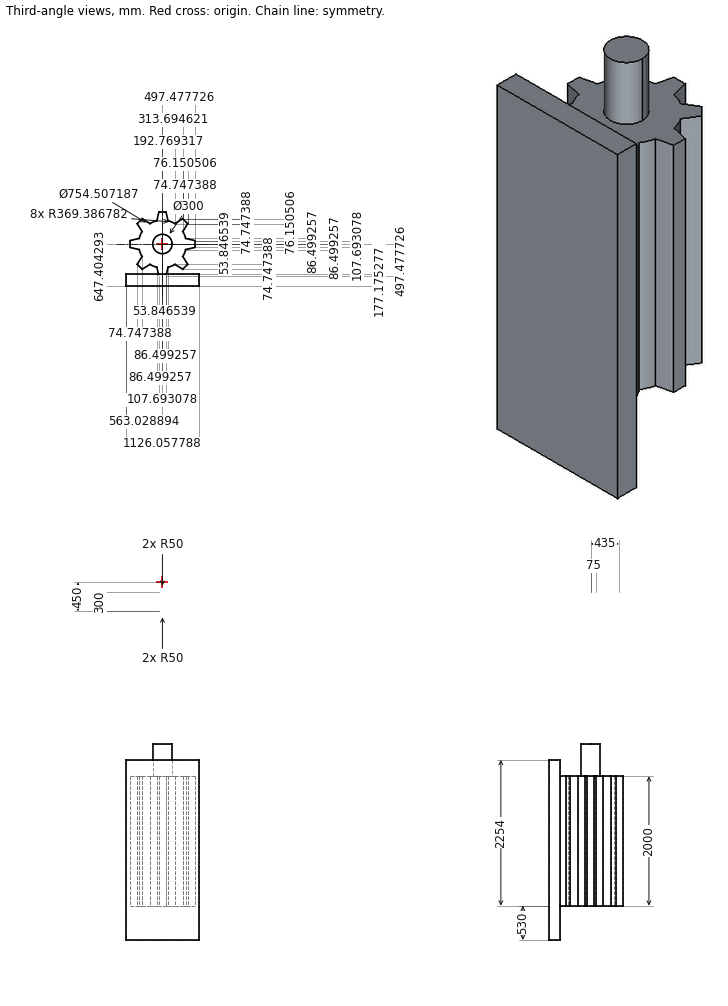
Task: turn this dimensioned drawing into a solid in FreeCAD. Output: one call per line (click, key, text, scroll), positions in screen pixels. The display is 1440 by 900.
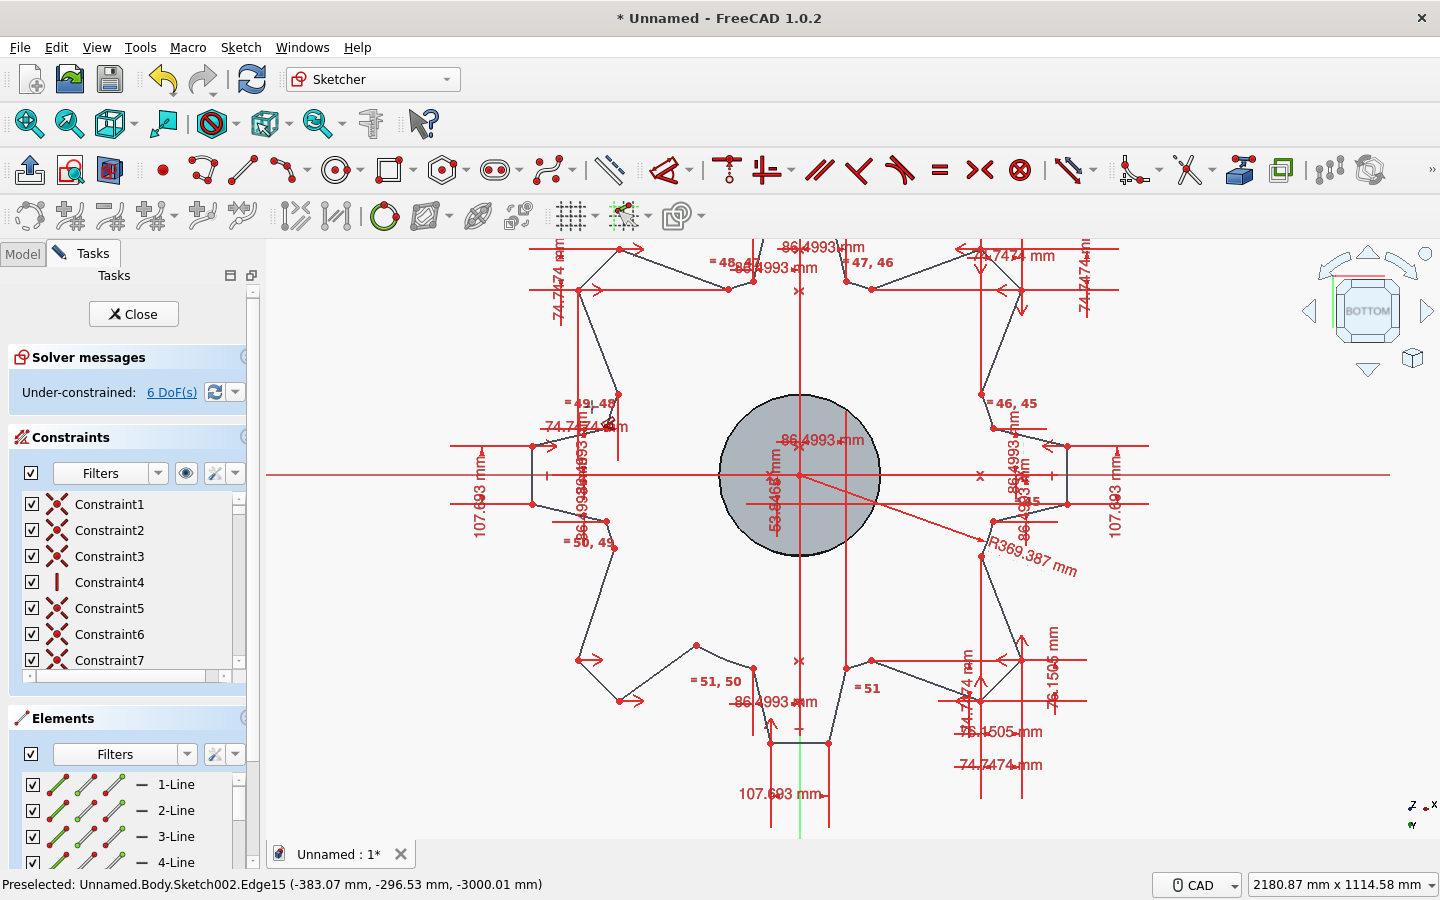
click(604, 582)
click(588, 694)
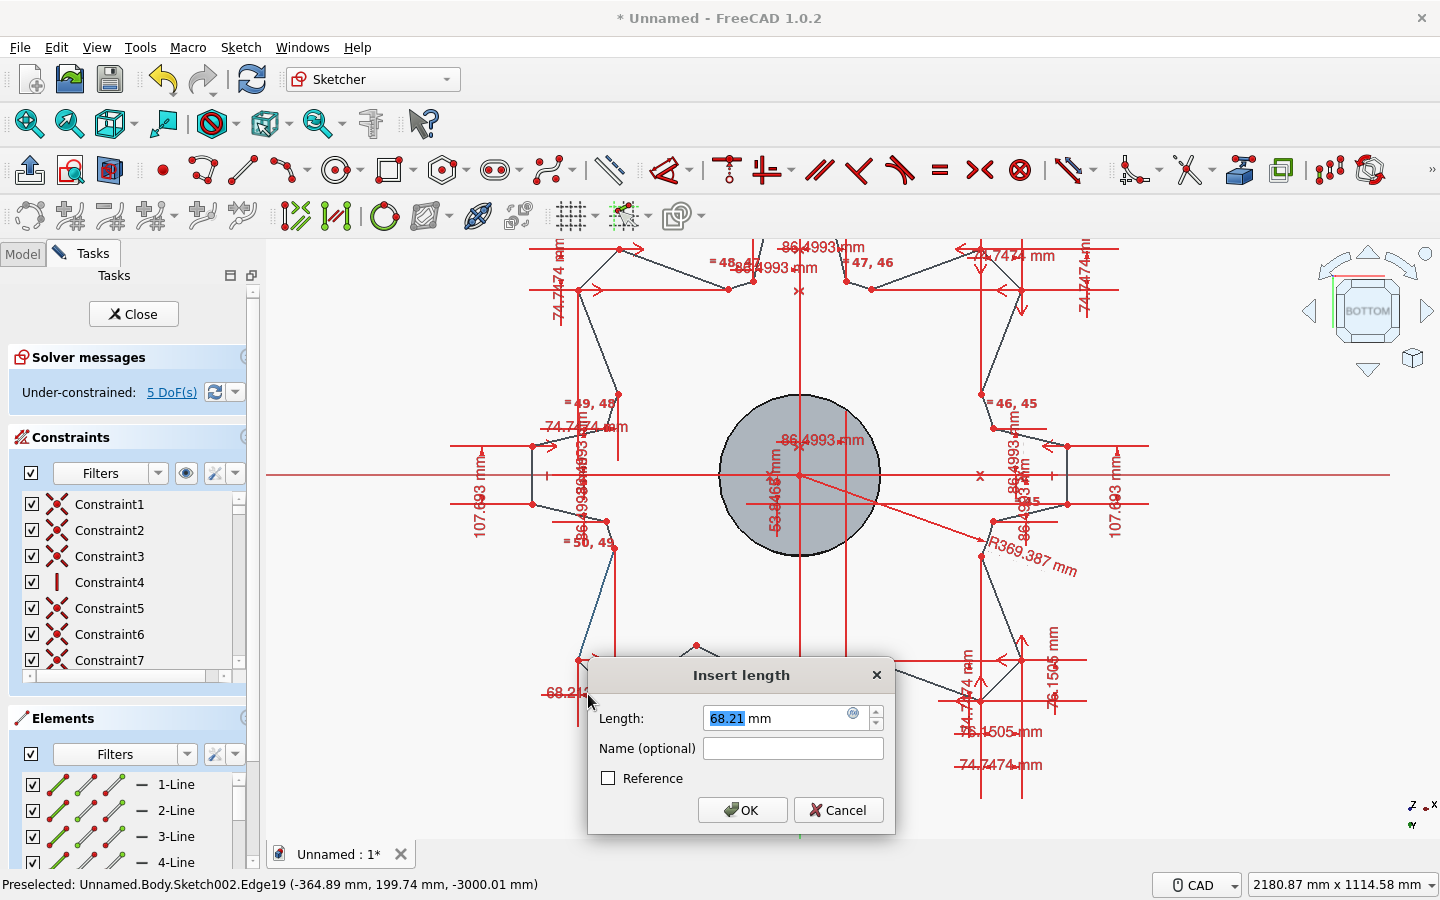
text(74.747388)
key(Return)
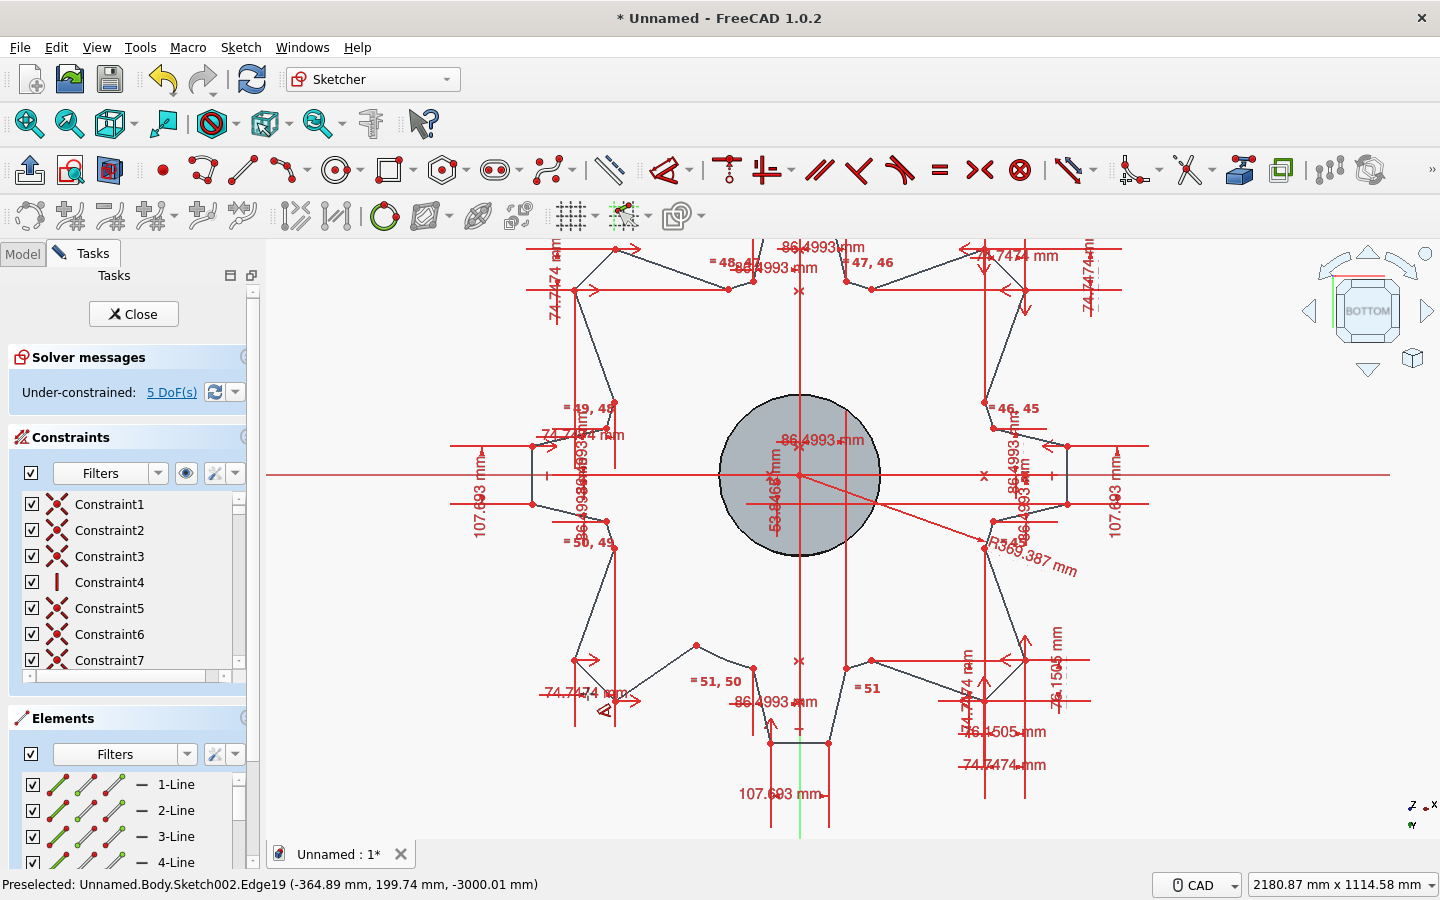
click(640, 684)
click(558, 673)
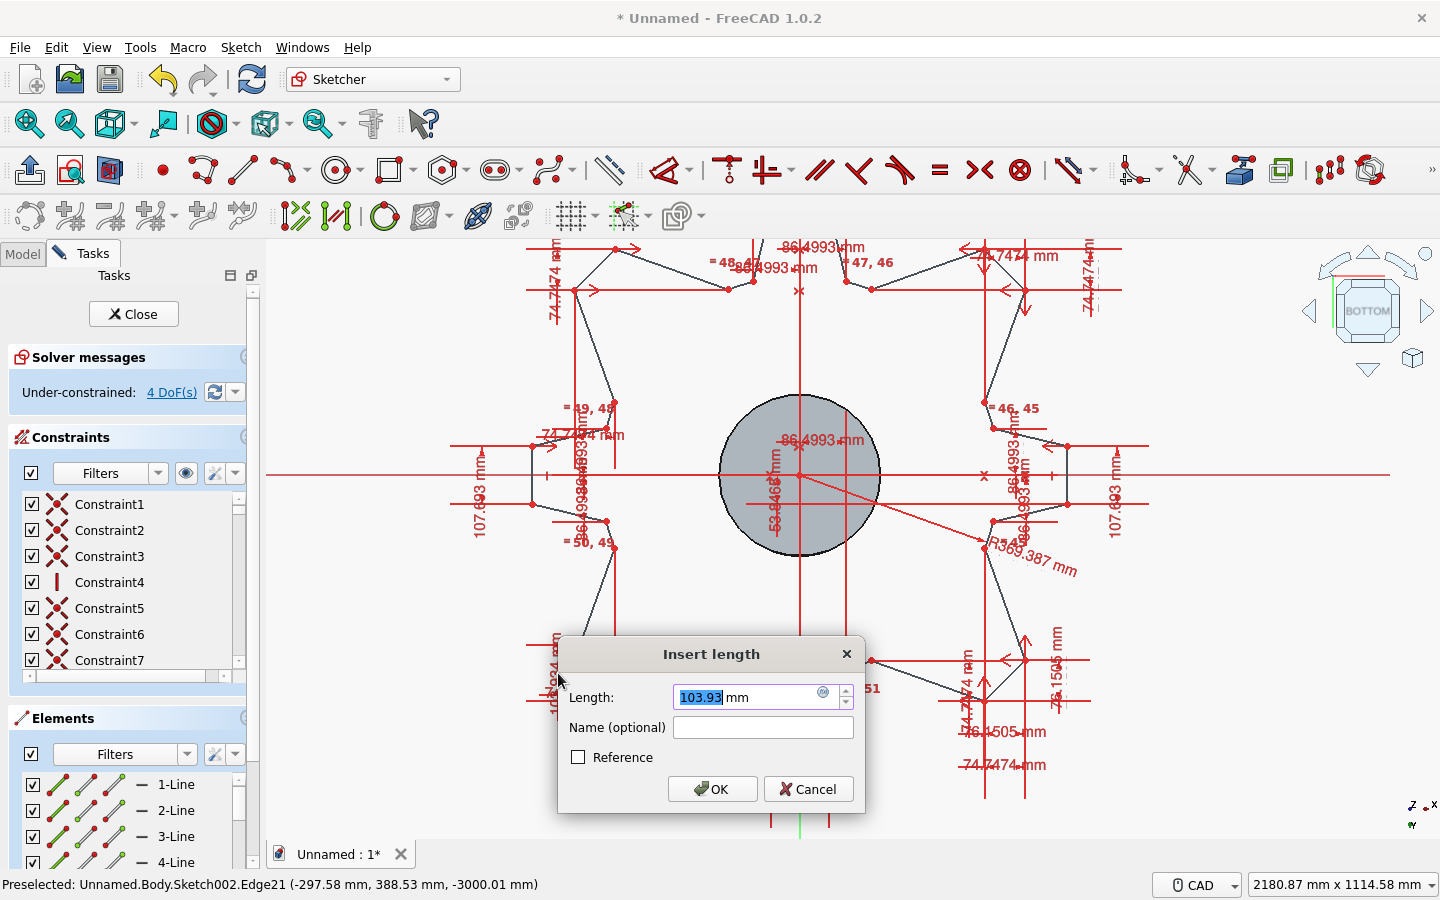
text(74.747388)
key(Return)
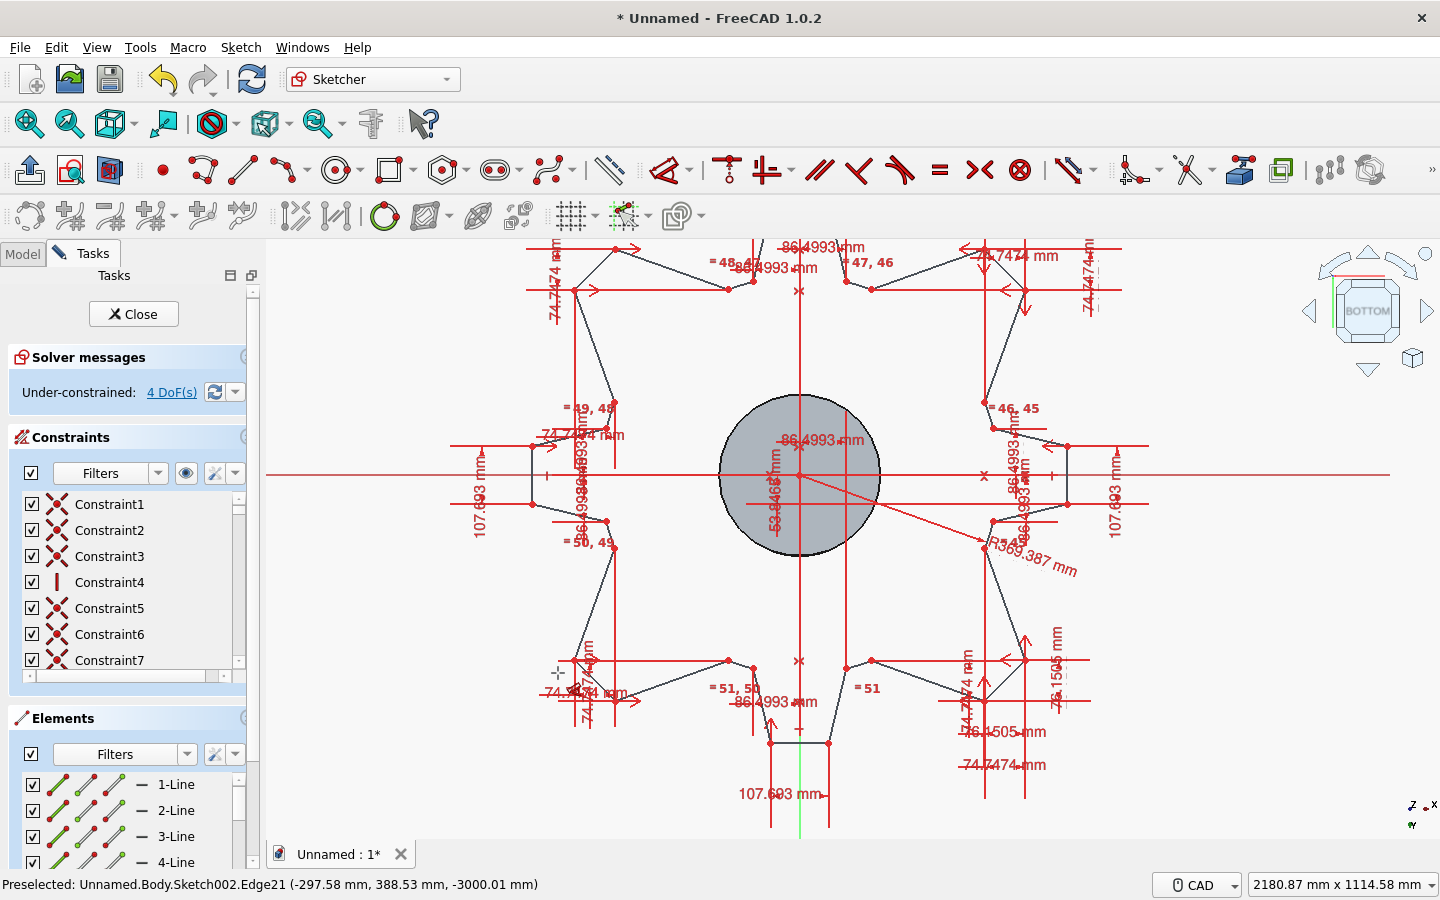
click(871, 661)
click(861, 695)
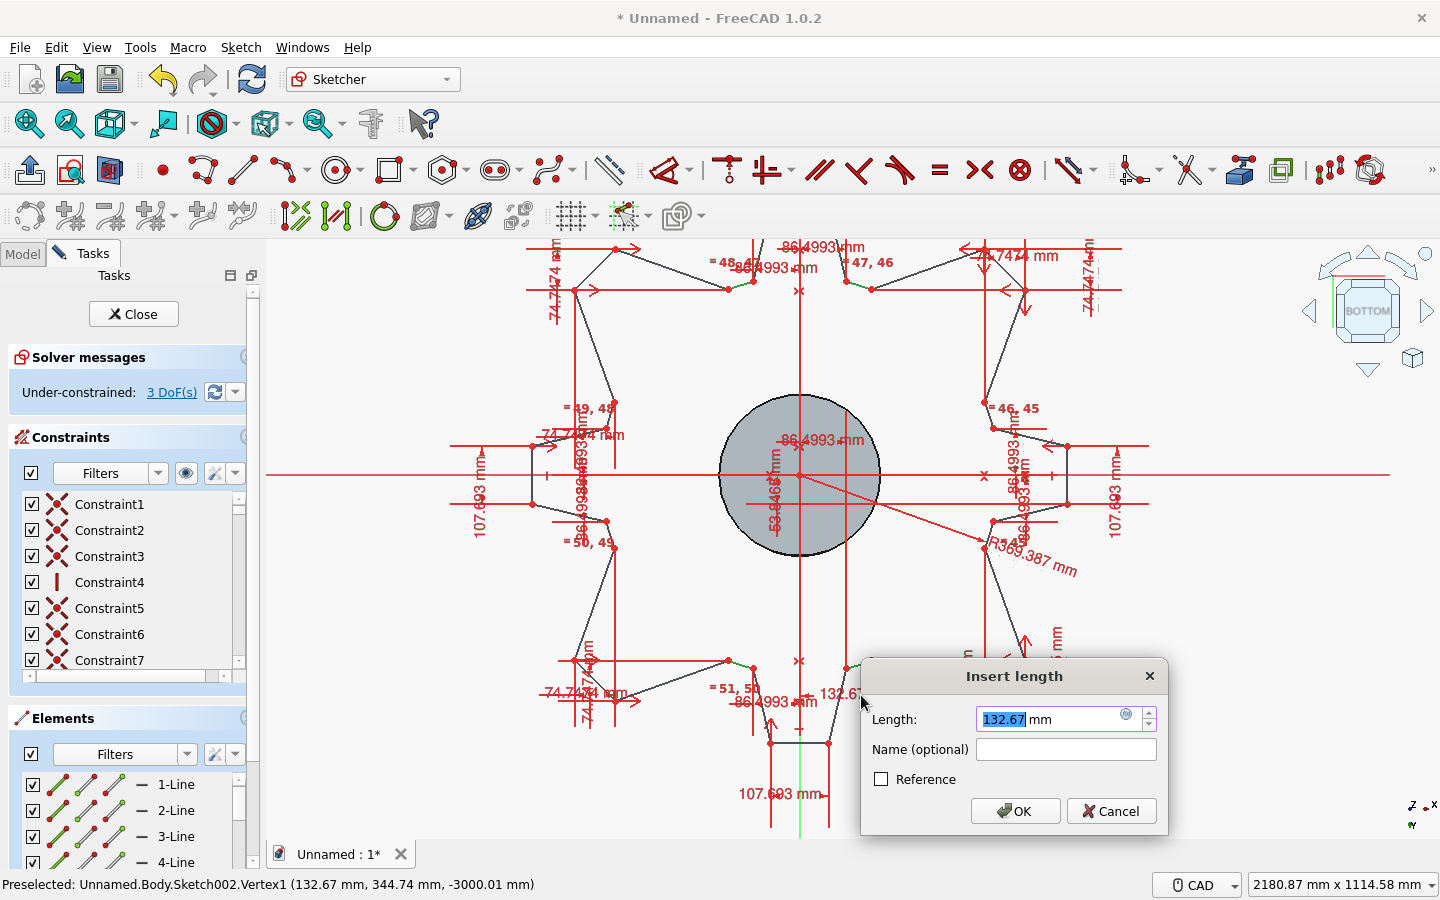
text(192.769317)
key(Return)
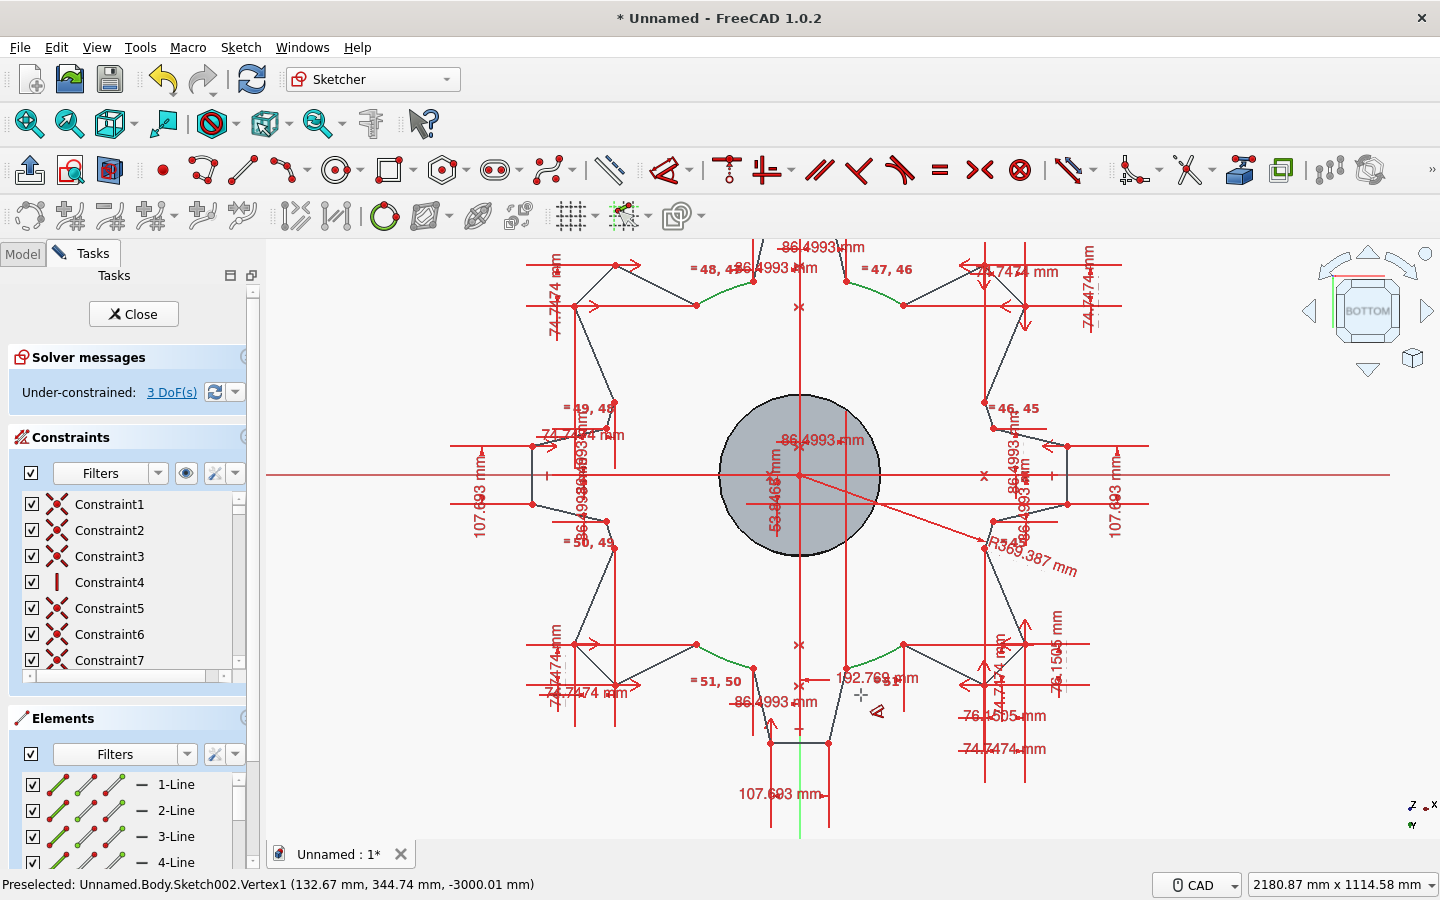
click(984, 685)
click(892, 719)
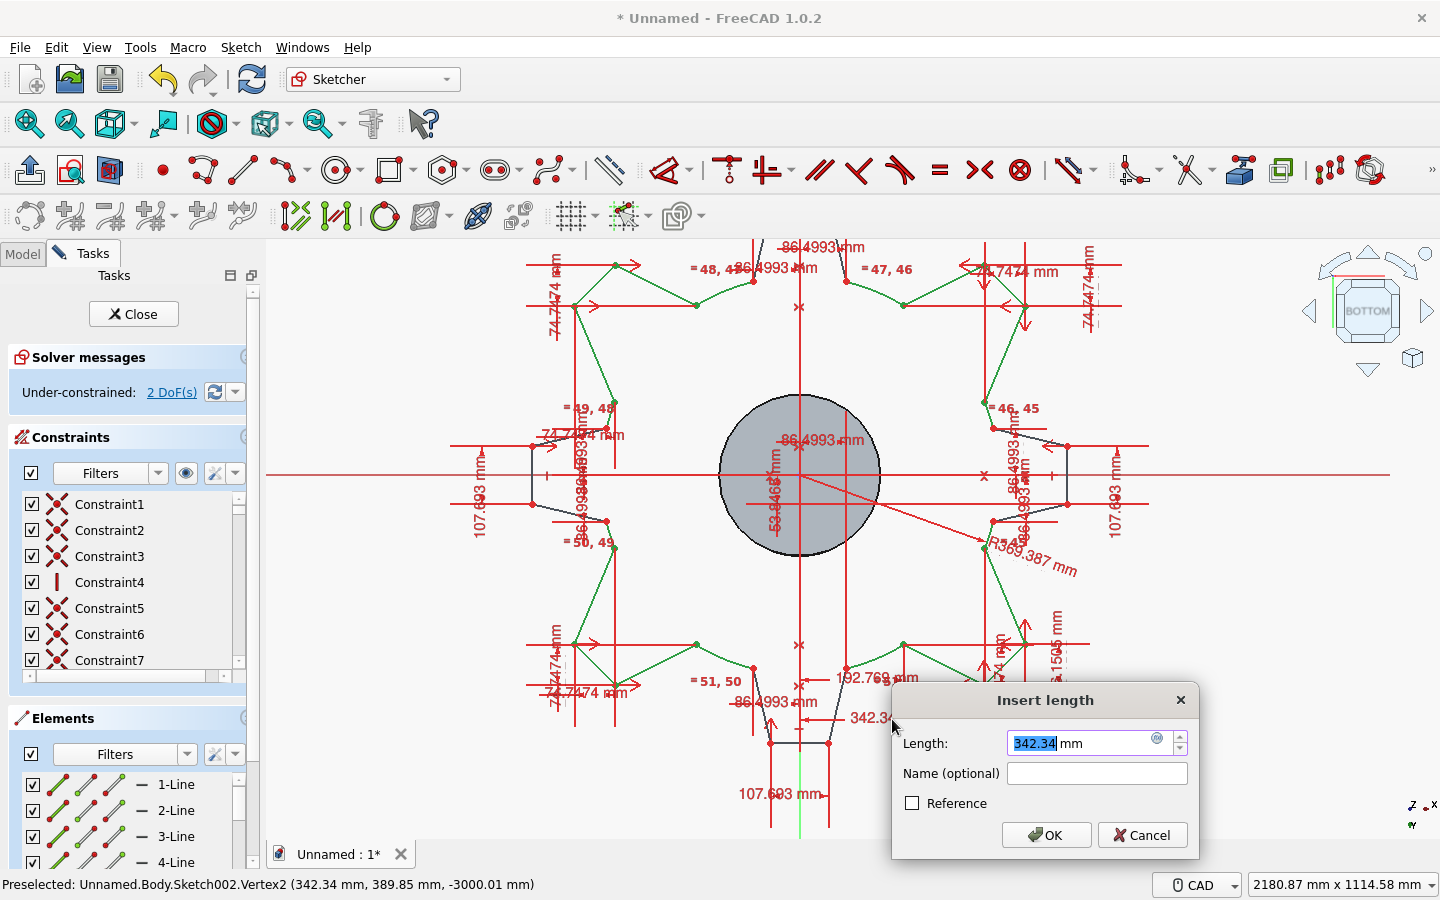
text(313.694621)
key(Return)